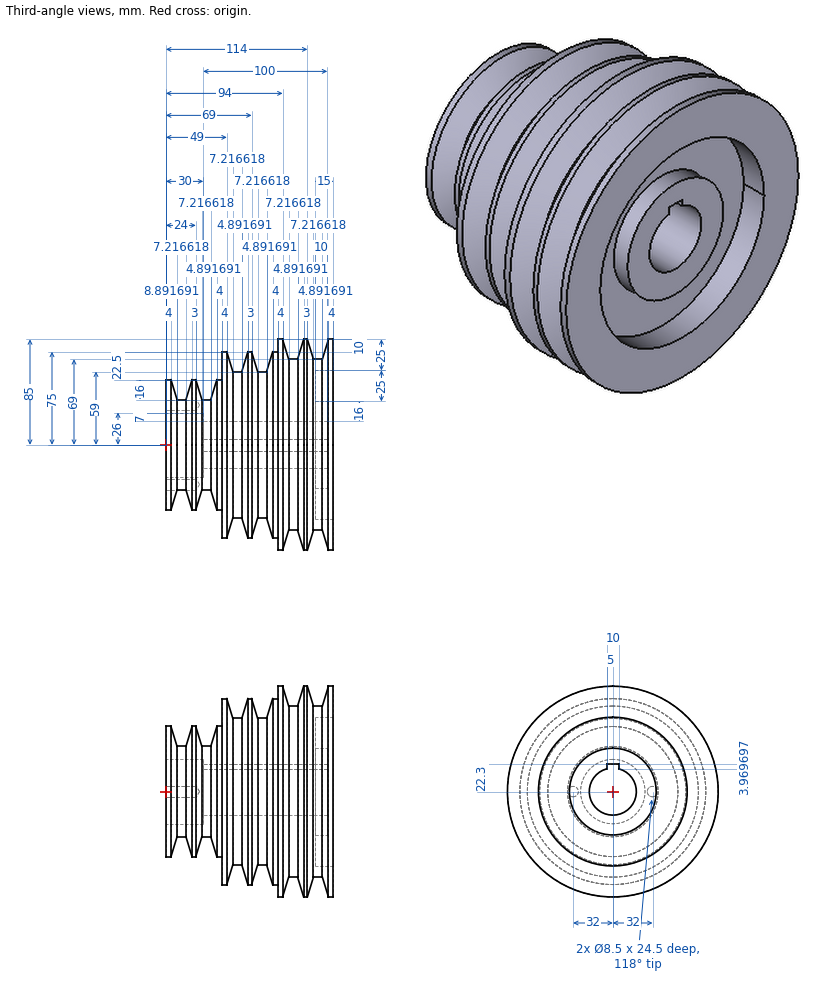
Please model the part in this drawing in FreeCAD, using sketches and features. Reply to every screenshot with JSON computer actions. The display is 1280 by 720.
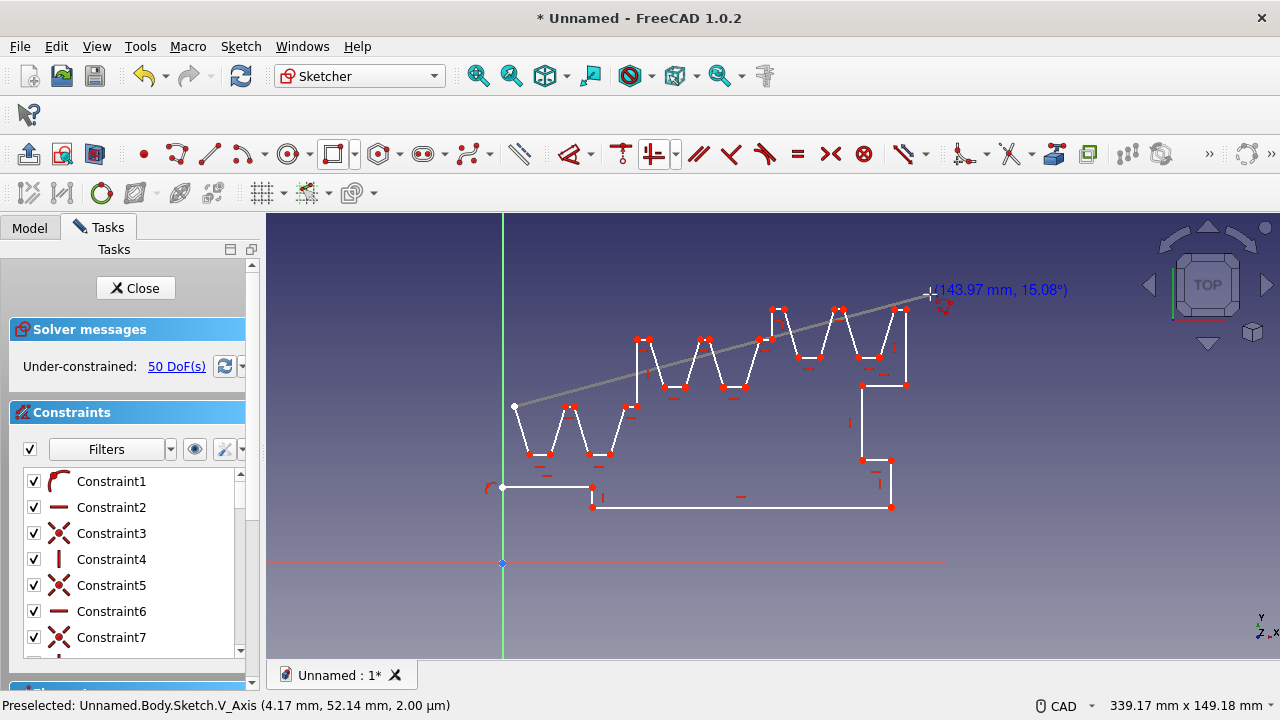
{"action": "scroll", "coordinate": [503, 406], "scroll_direction": "up", "scroll_amount": 2}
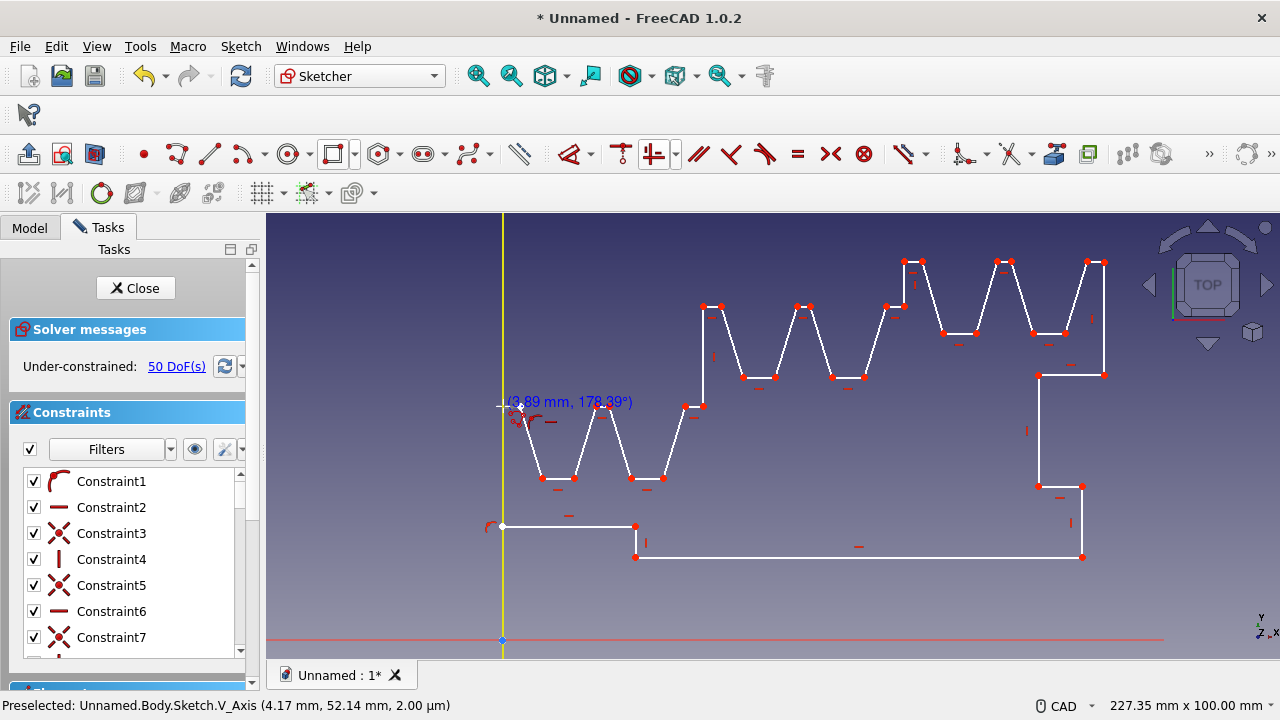
{"action": "left_click", "coordinate": [512, 406]}
{"action": "left_click", "coordinate": [503, 527]}
{"action": "key", "text": "Escape"}
{"action": "key", "text": "Escape"}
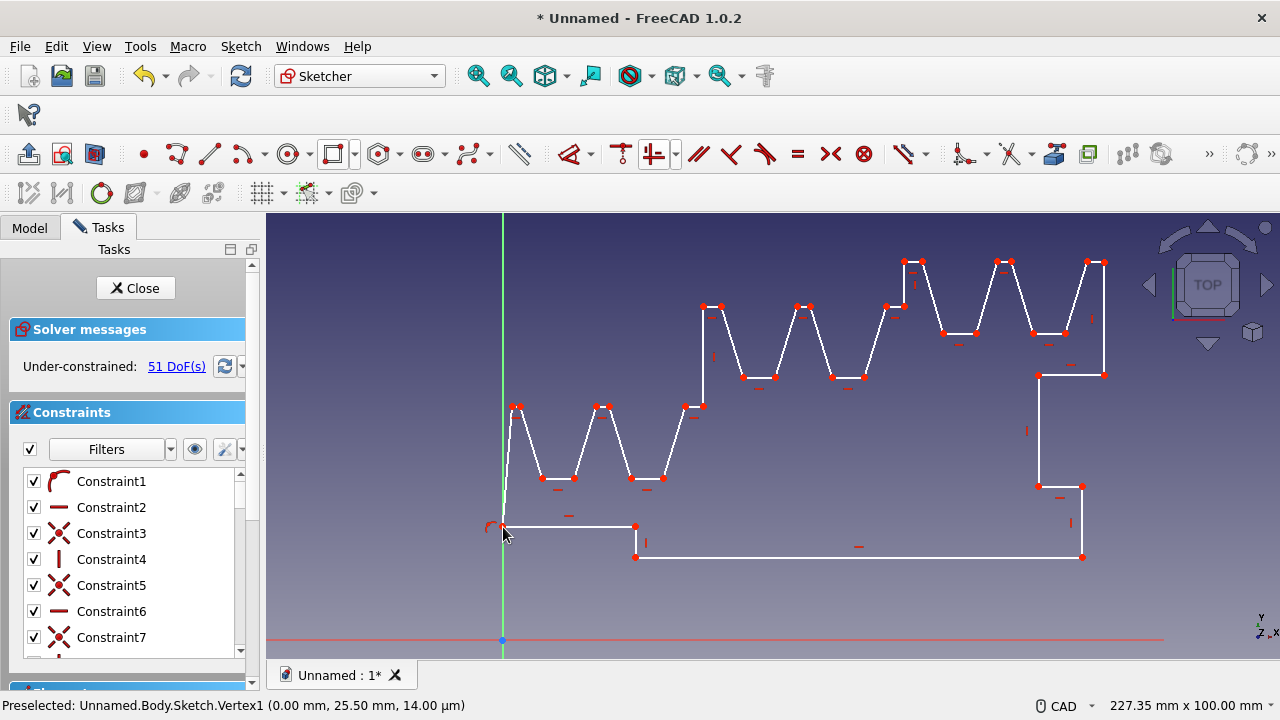
{"action": "scroll", "coordinate": [1096, 262], "scroll_direction": "up", "scroll_amount": 3}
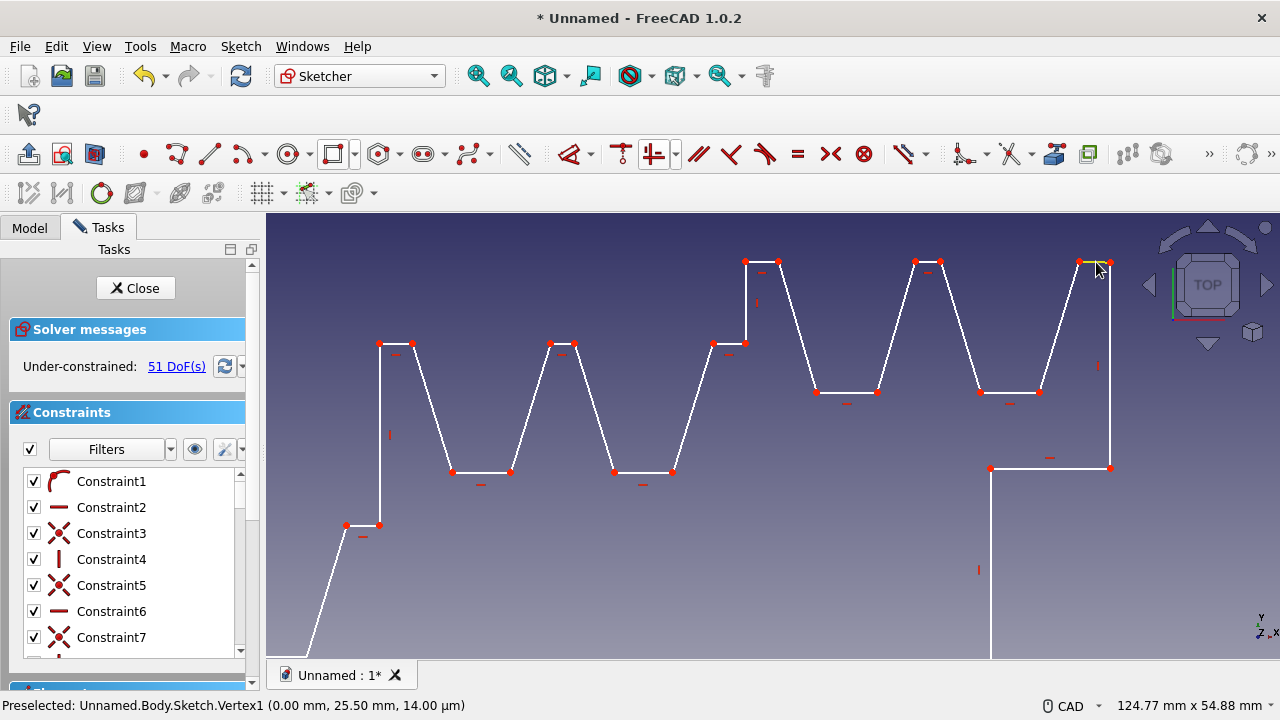
{"action": "left_click", "coordinate": [1095, 262]}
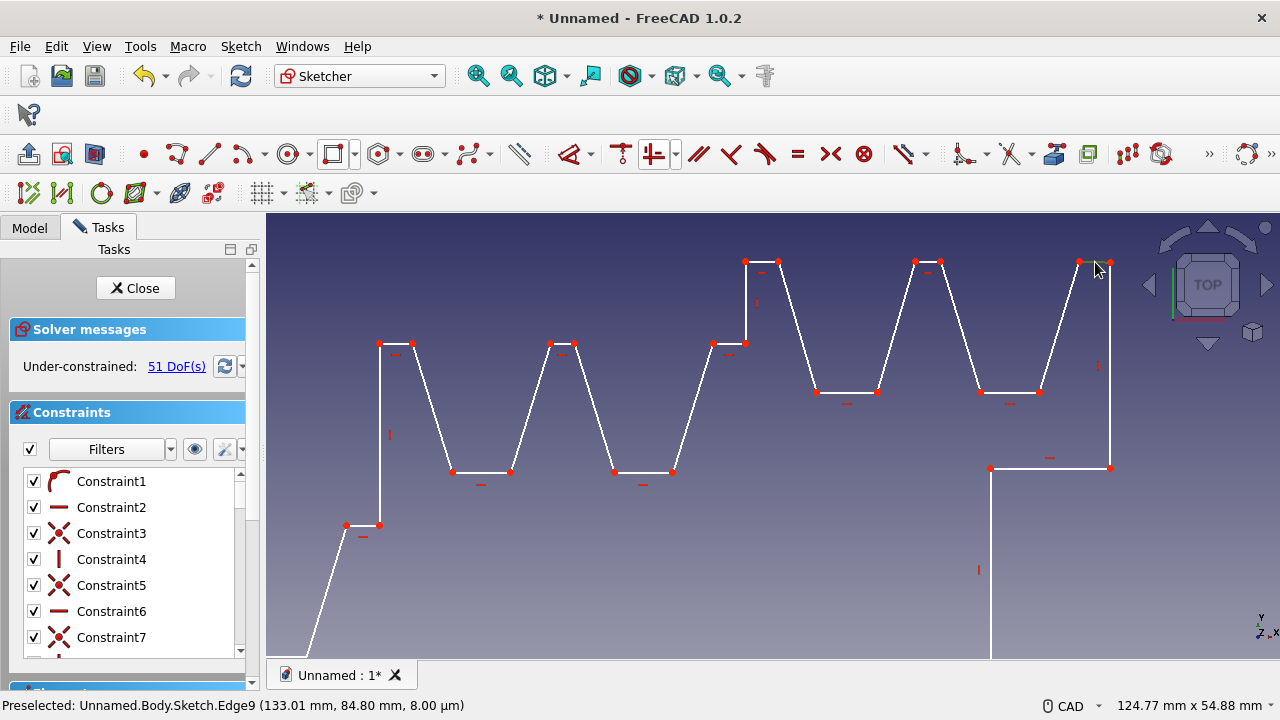
{"action": "key", "text": "h"}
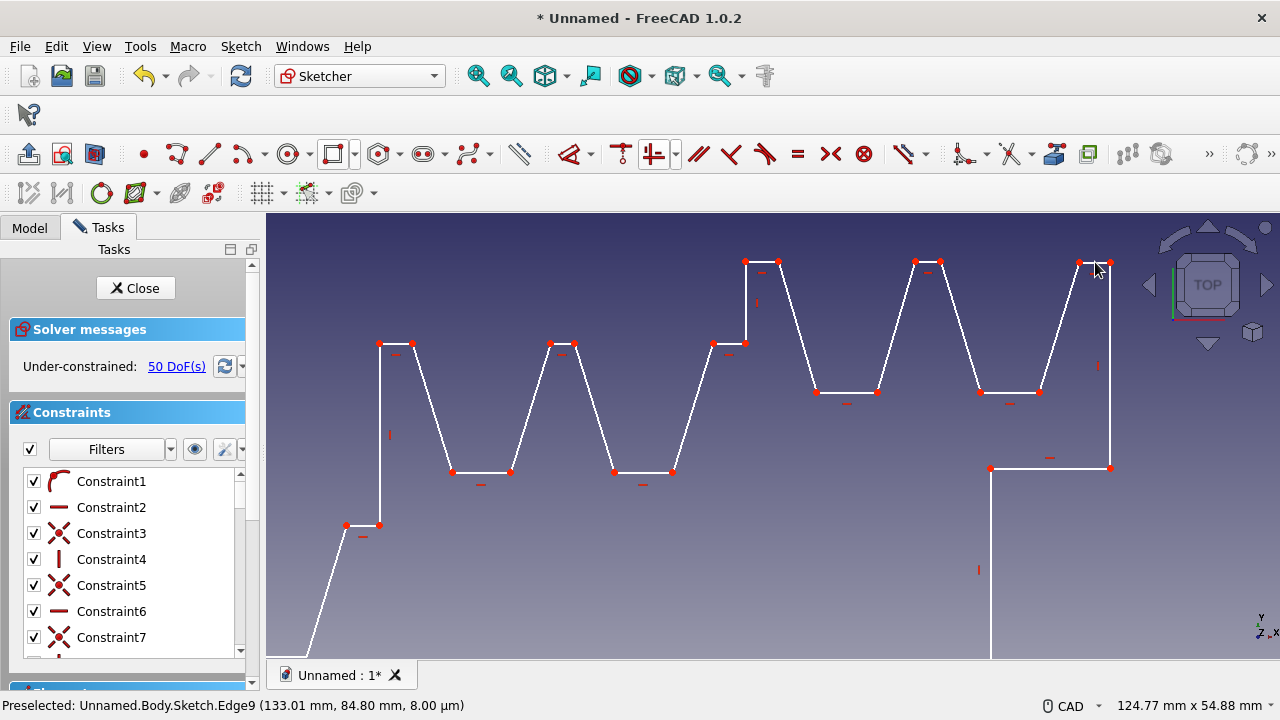
{"action": "scroll", "coordinate": [787, 337], "scroll_direction": "down", "scroll_amount": 5}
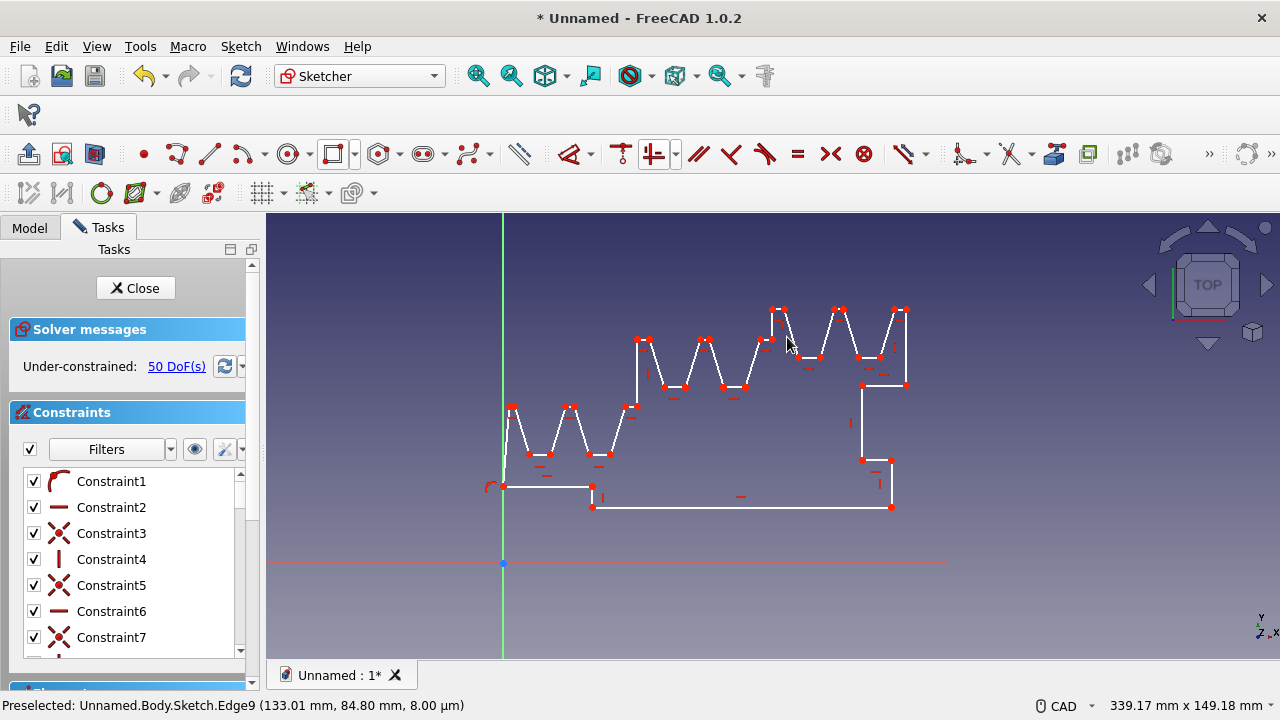
{"action": "scroll", "coordinate": [507, 431], "scroll_direction": "up", "scroll_amount": 6}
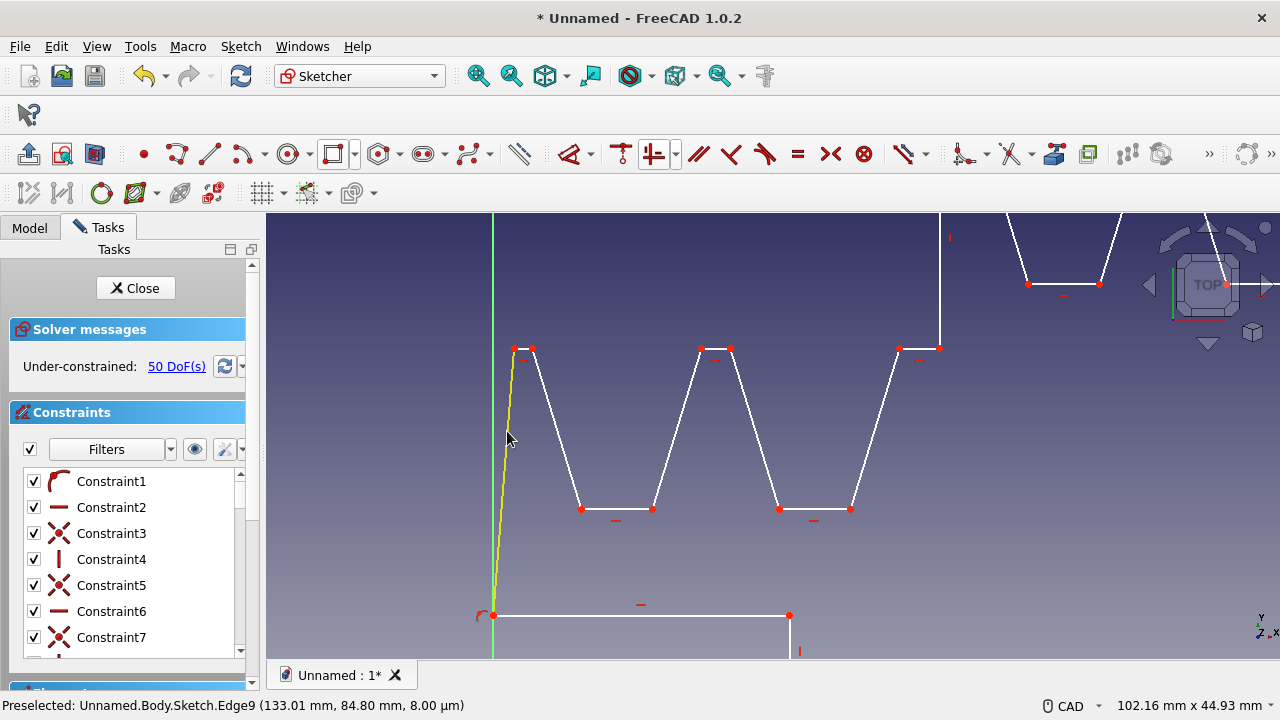
{"action": "left_click", "coordinate": [508, 429]}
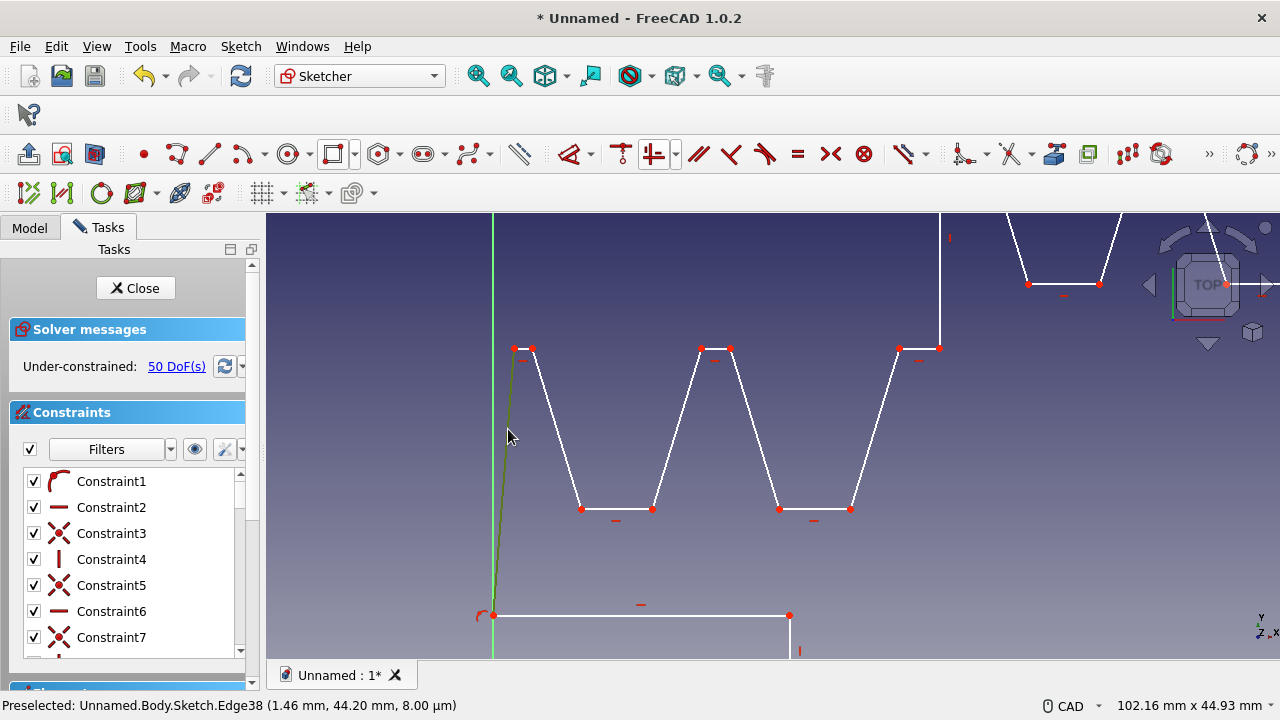
{"action": "left_click", "coordinate": [676, 154]}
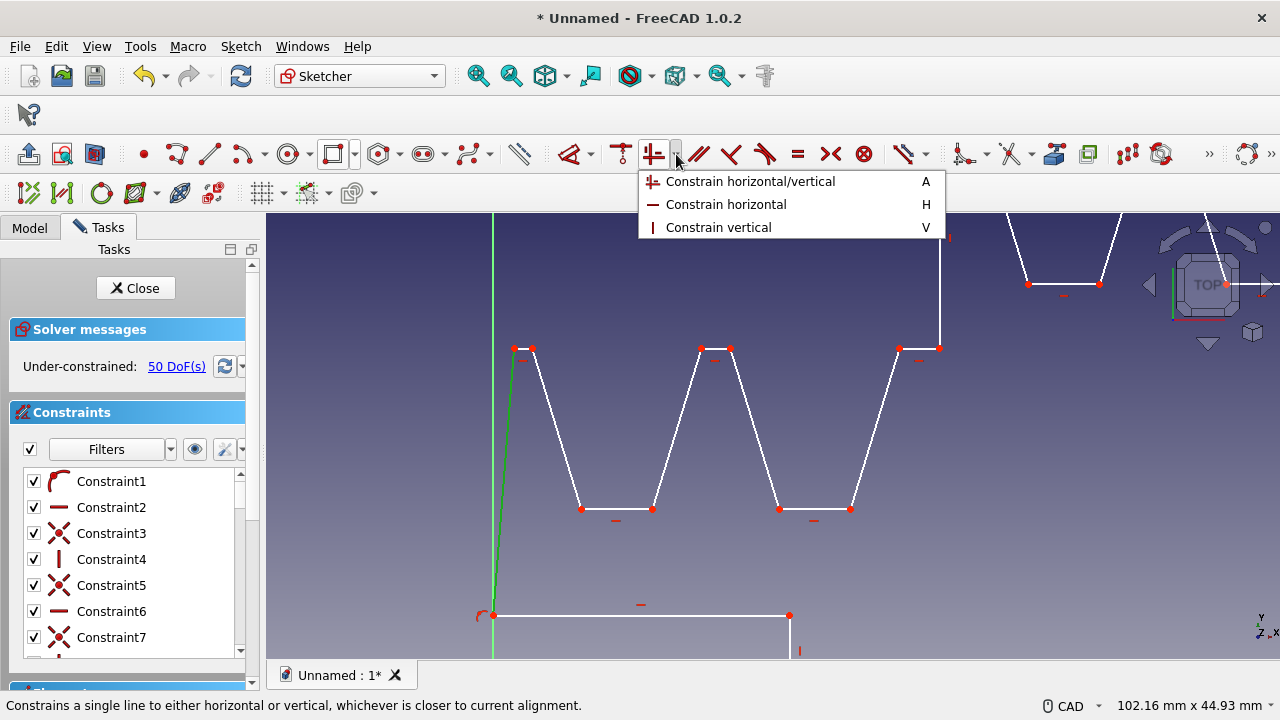
{"action": "left_click", "coordinate": [792, 228]}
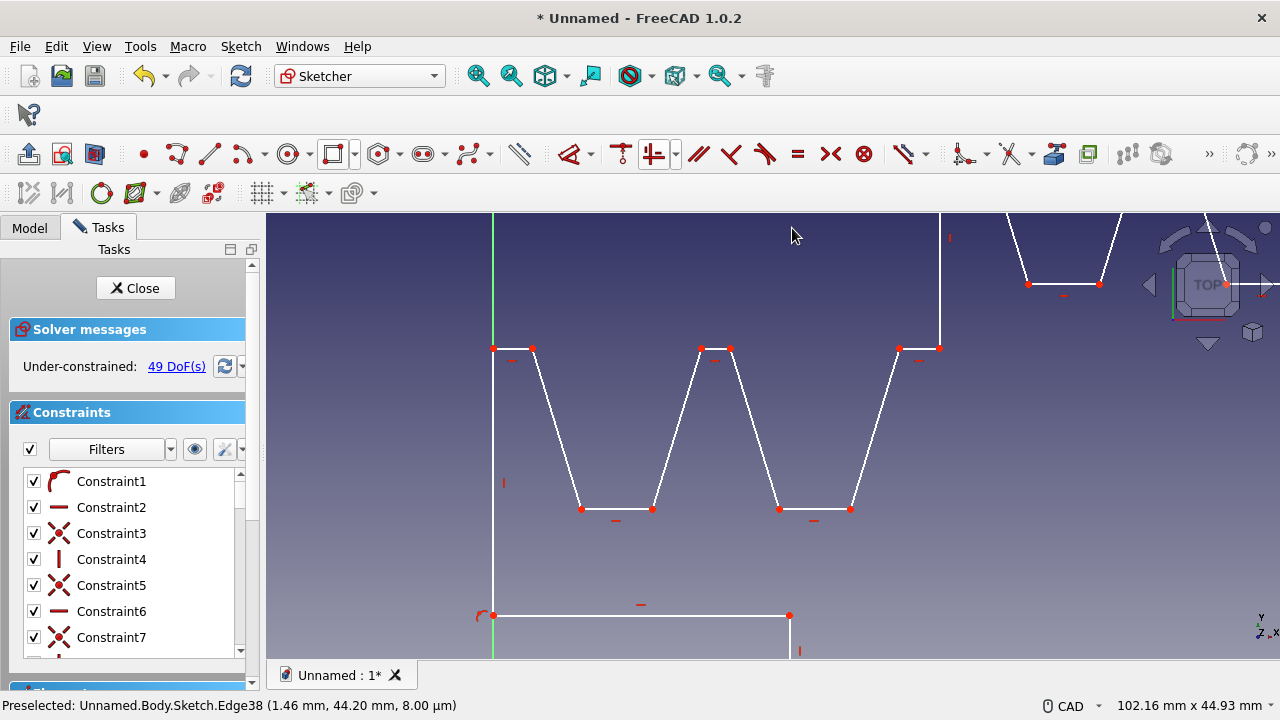
{"action": "left_click", "coordinate": [568, 154]}